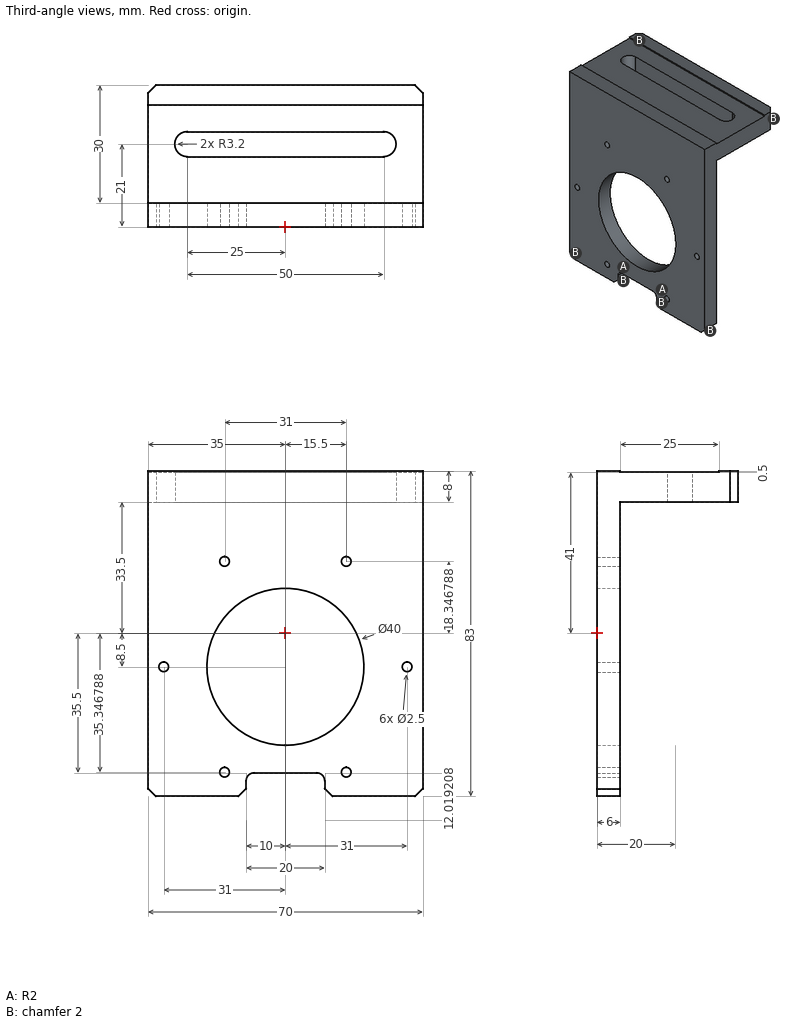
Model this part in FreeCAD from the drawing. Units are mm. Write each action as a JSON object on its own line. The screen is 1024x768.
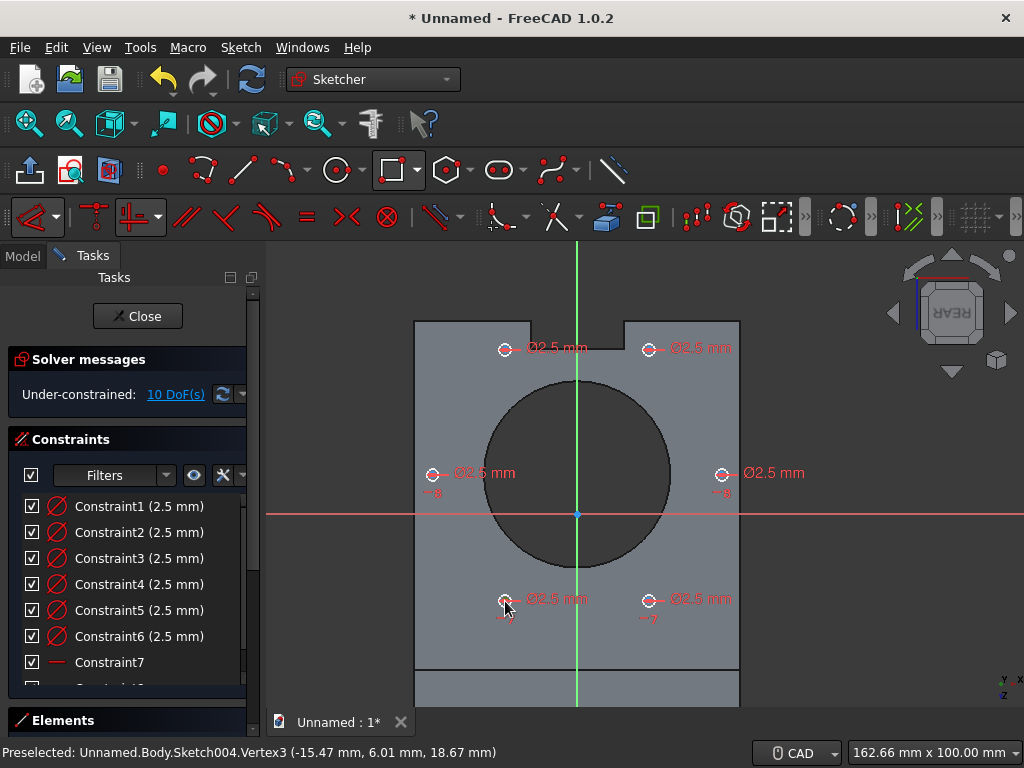
{"action": "left_click", "coordinate": [505, 350]}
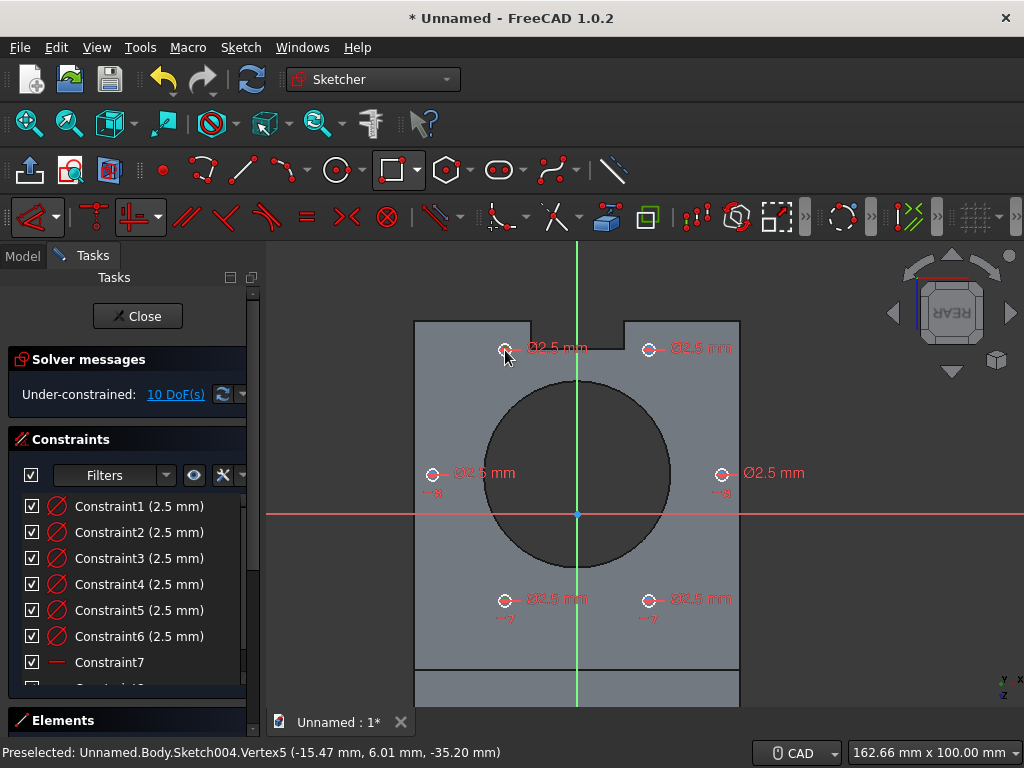
{"action": "left_click", "coordinate": [160, 218]}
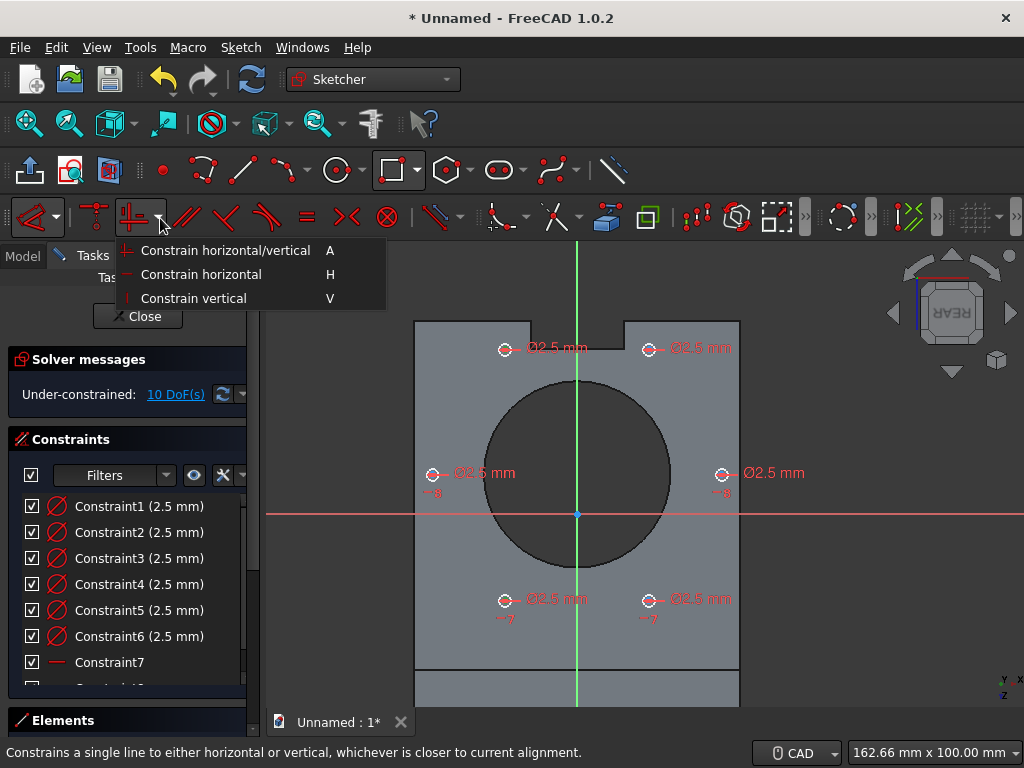
{"action": "left_click", "coordinate": [251, 298]}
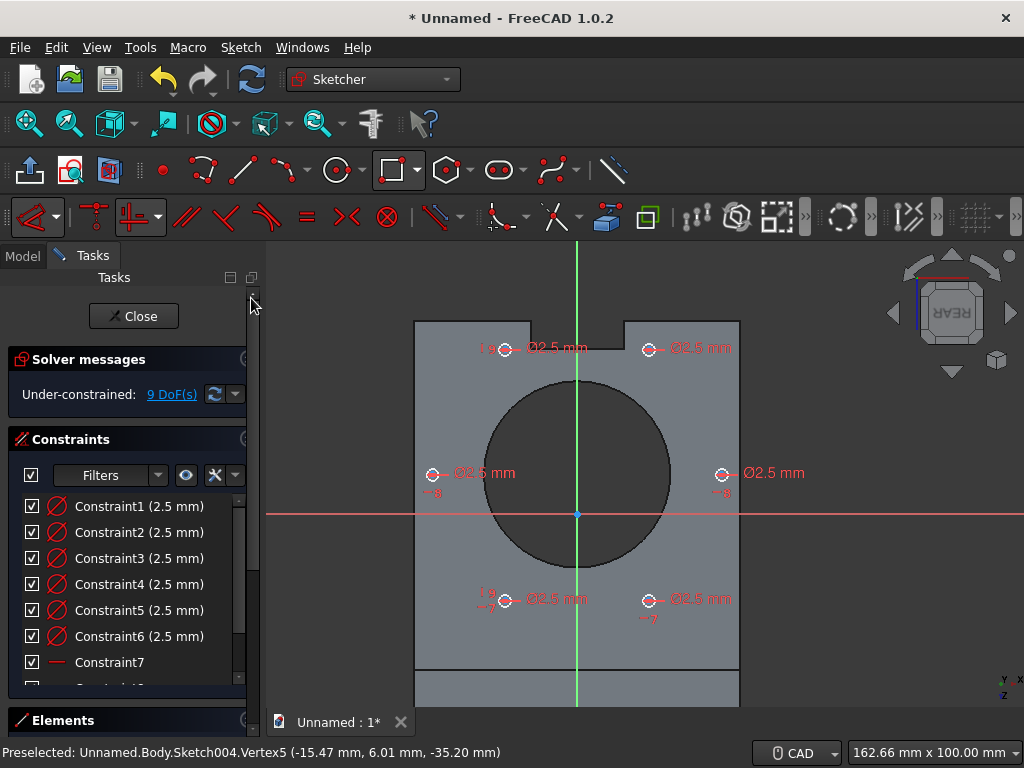
{"action": "left_click", "coordinate": [649, 601]}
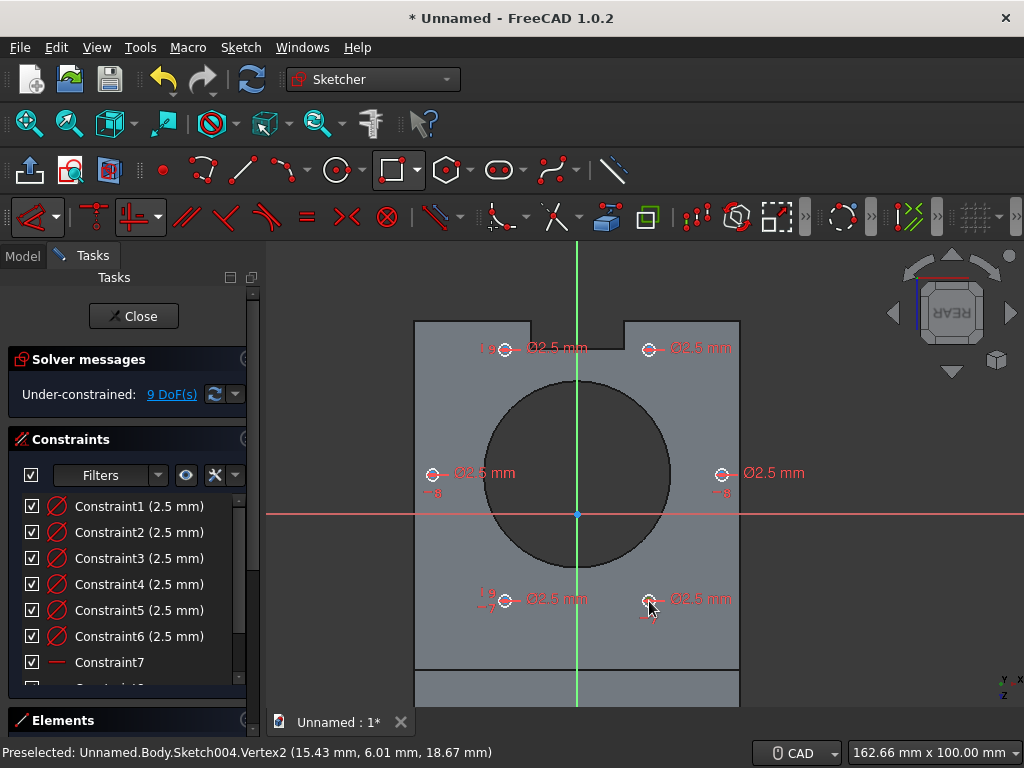
{"action": "left_click", "coordinate": [649, 350]}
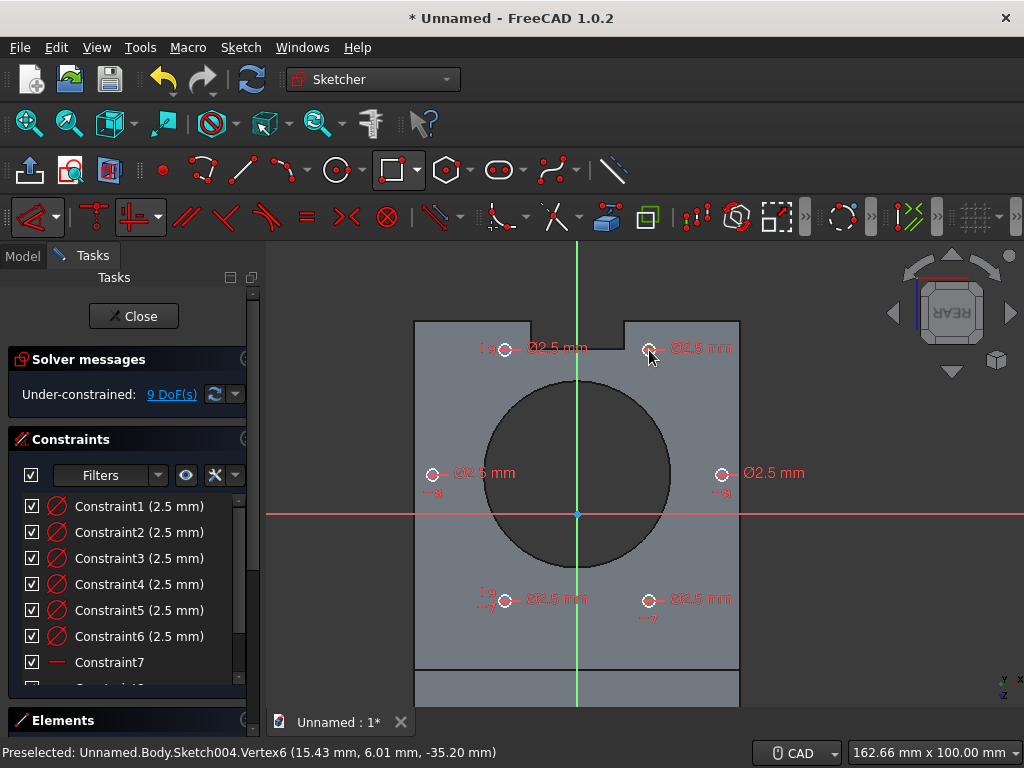
{"action": "left_click", "coordinate": [160, 218]}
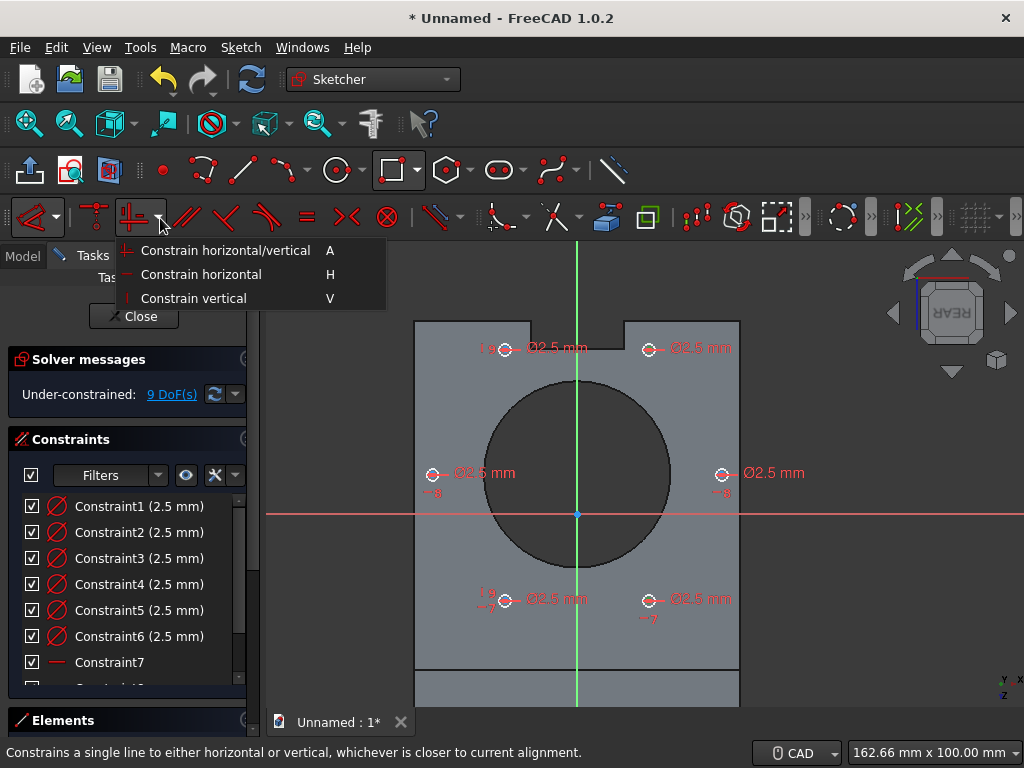
{"action": "left_click", "coordinate": [251, 298]}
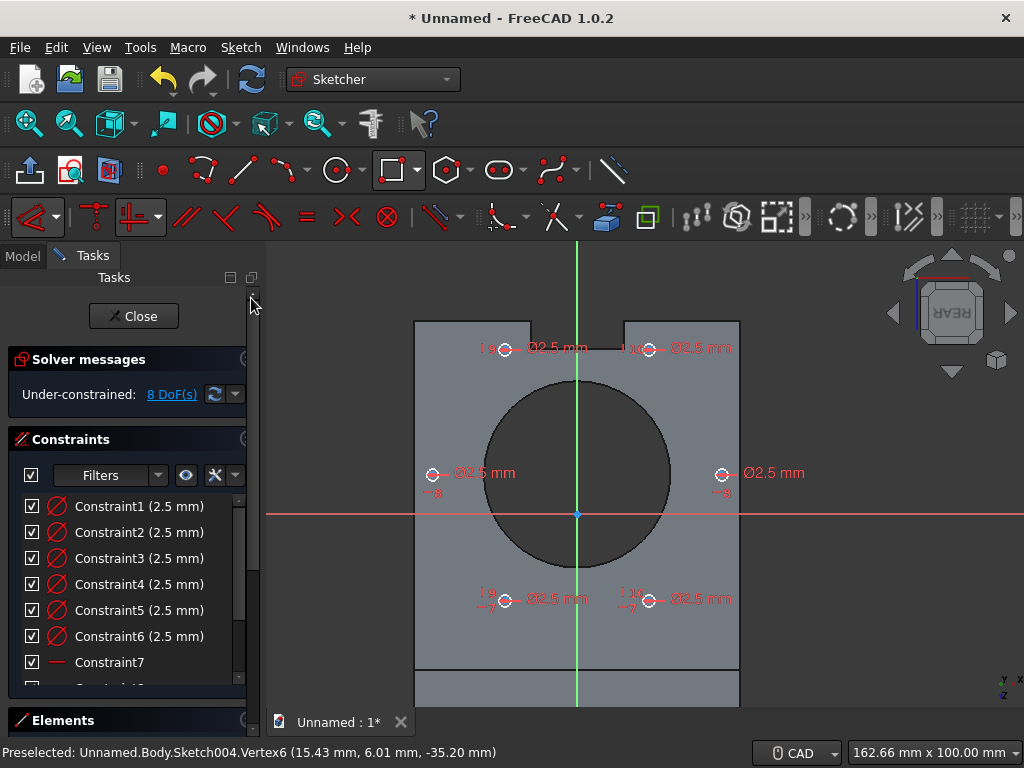
{"action": "left_click", "coordinate": [505, 350]}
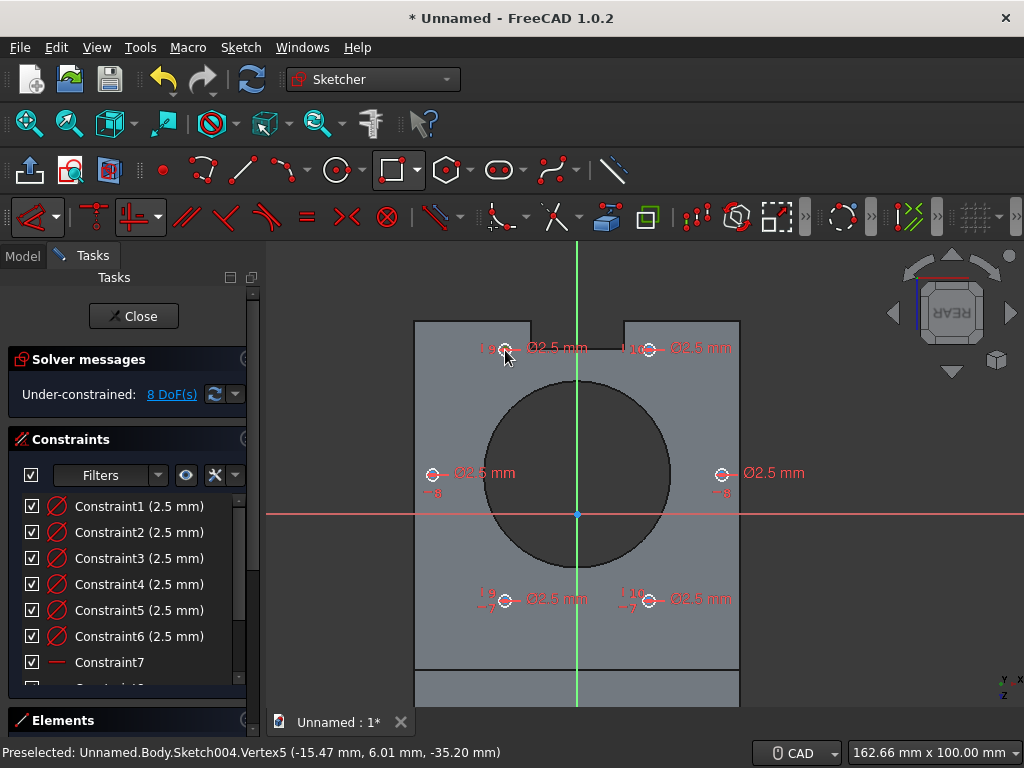
{"action": "left_click", "coordinate": [649, 350]}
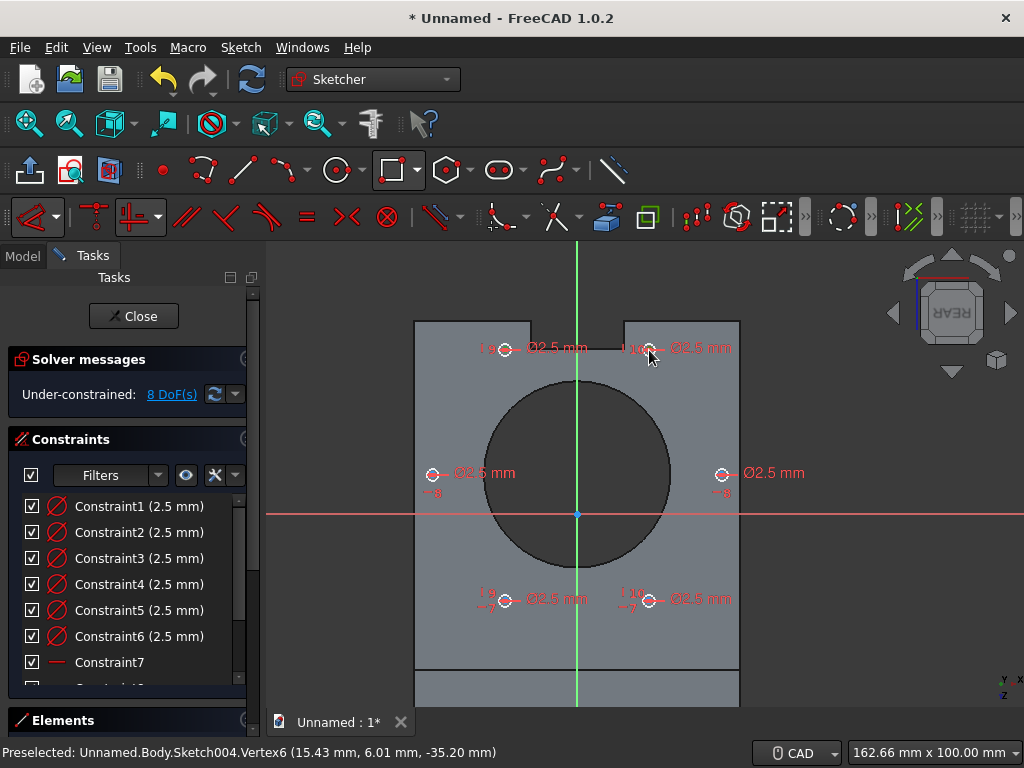
{"action": "key", "text": "h"}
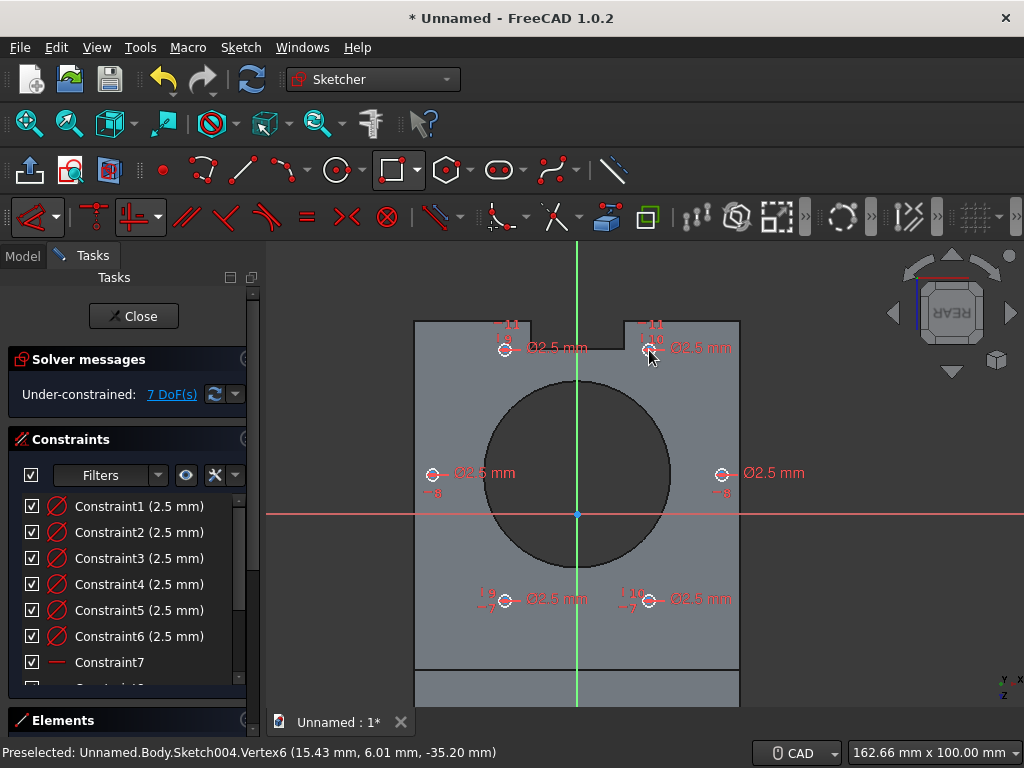
{"action": "left_click", "coordinate": [722, 475]}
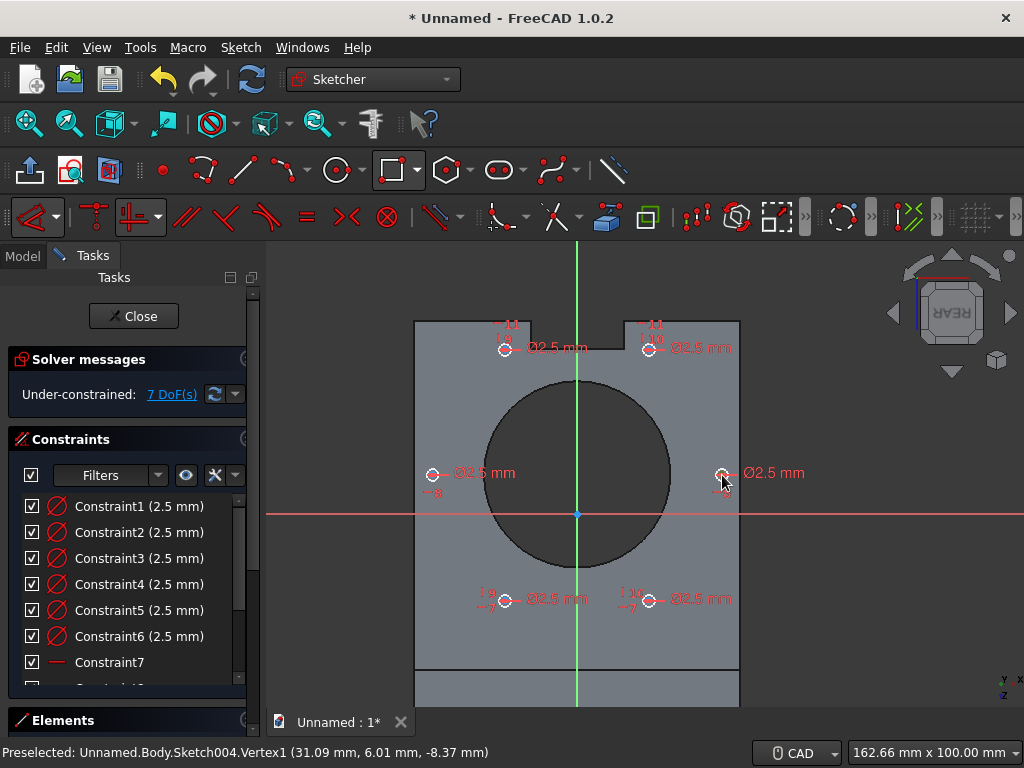
{"action": "left_click", "coordinate": [58, 218]}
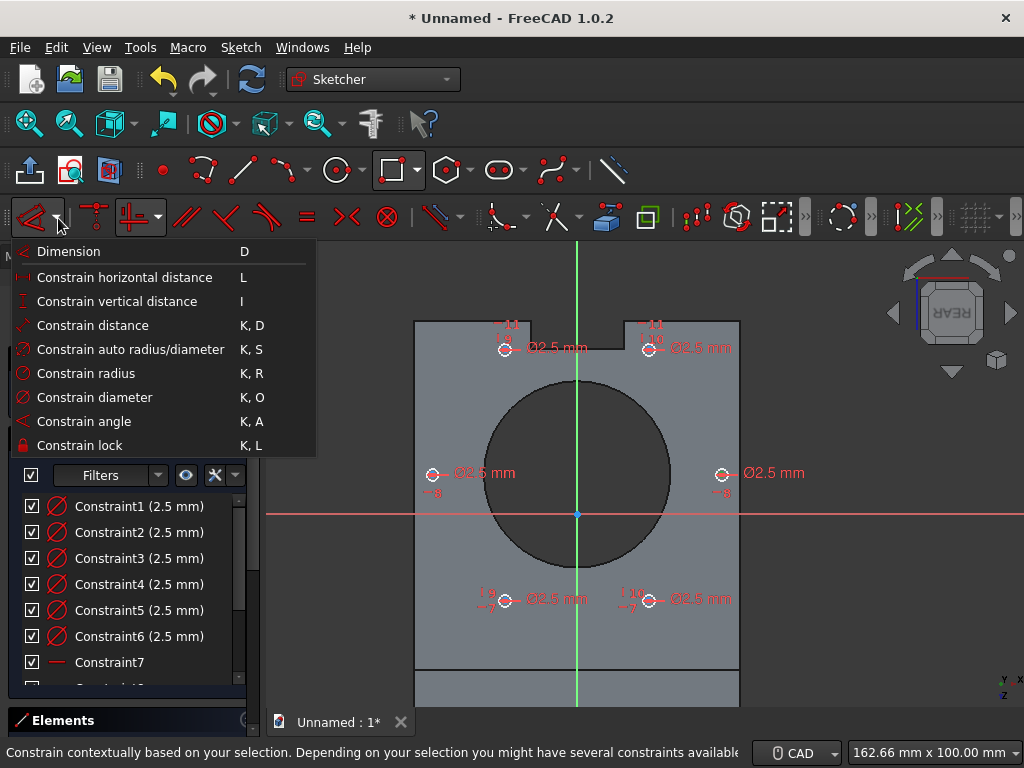
{"action": "left_click", "coordinate": [164, 277]}